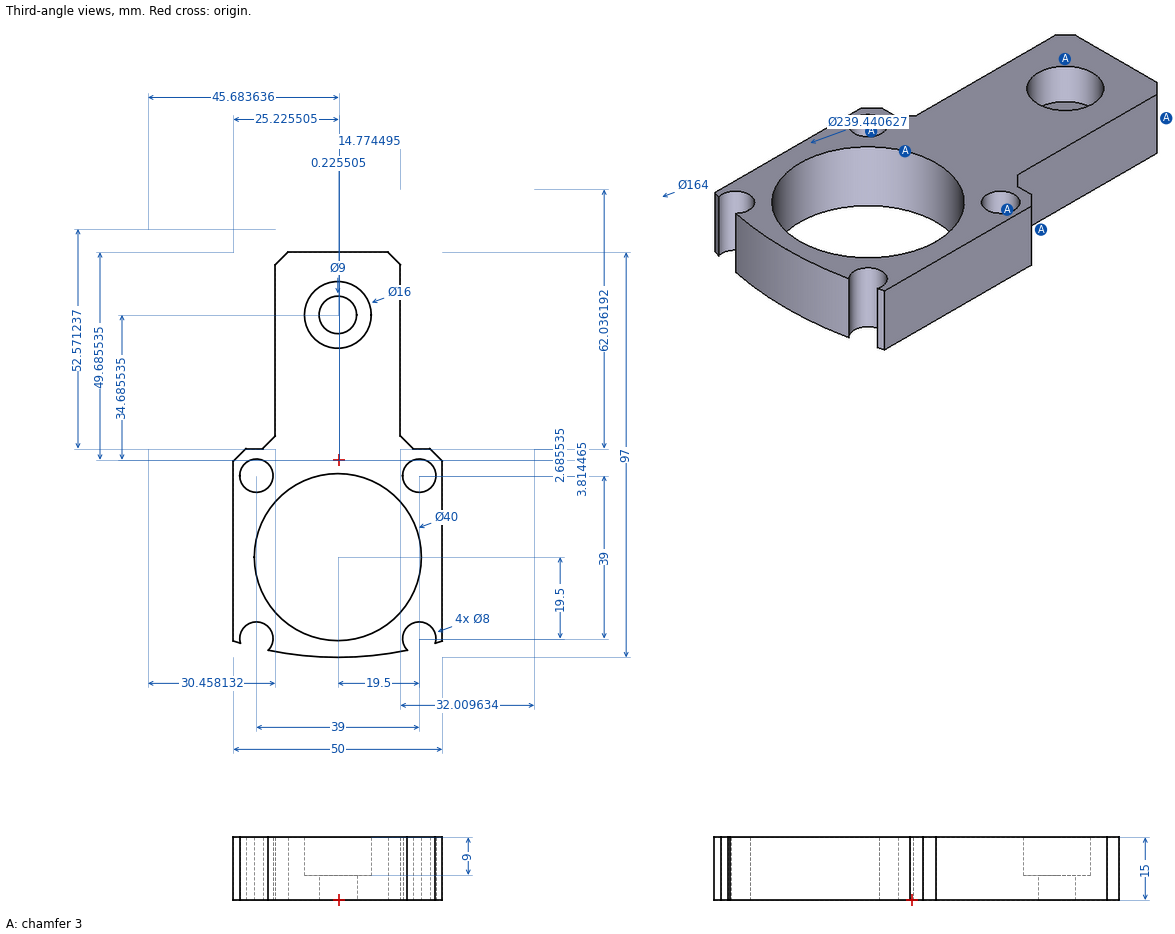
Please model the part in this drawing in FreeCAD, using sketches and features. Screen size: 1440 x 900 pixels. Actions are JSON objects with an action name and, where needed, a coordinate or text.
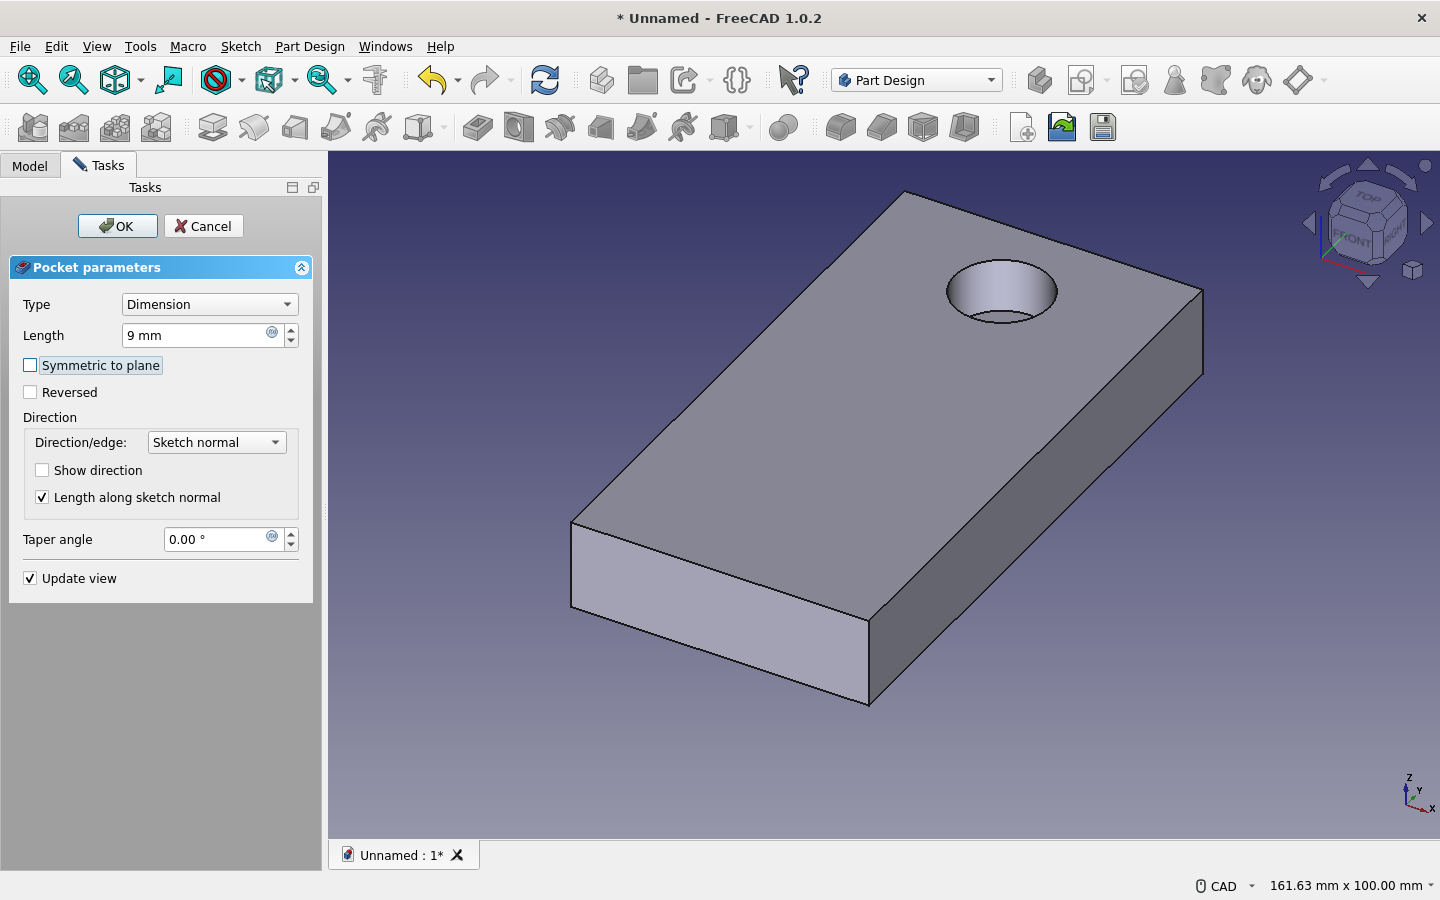
{"action": "left_click", "coordinate": [118, 226]}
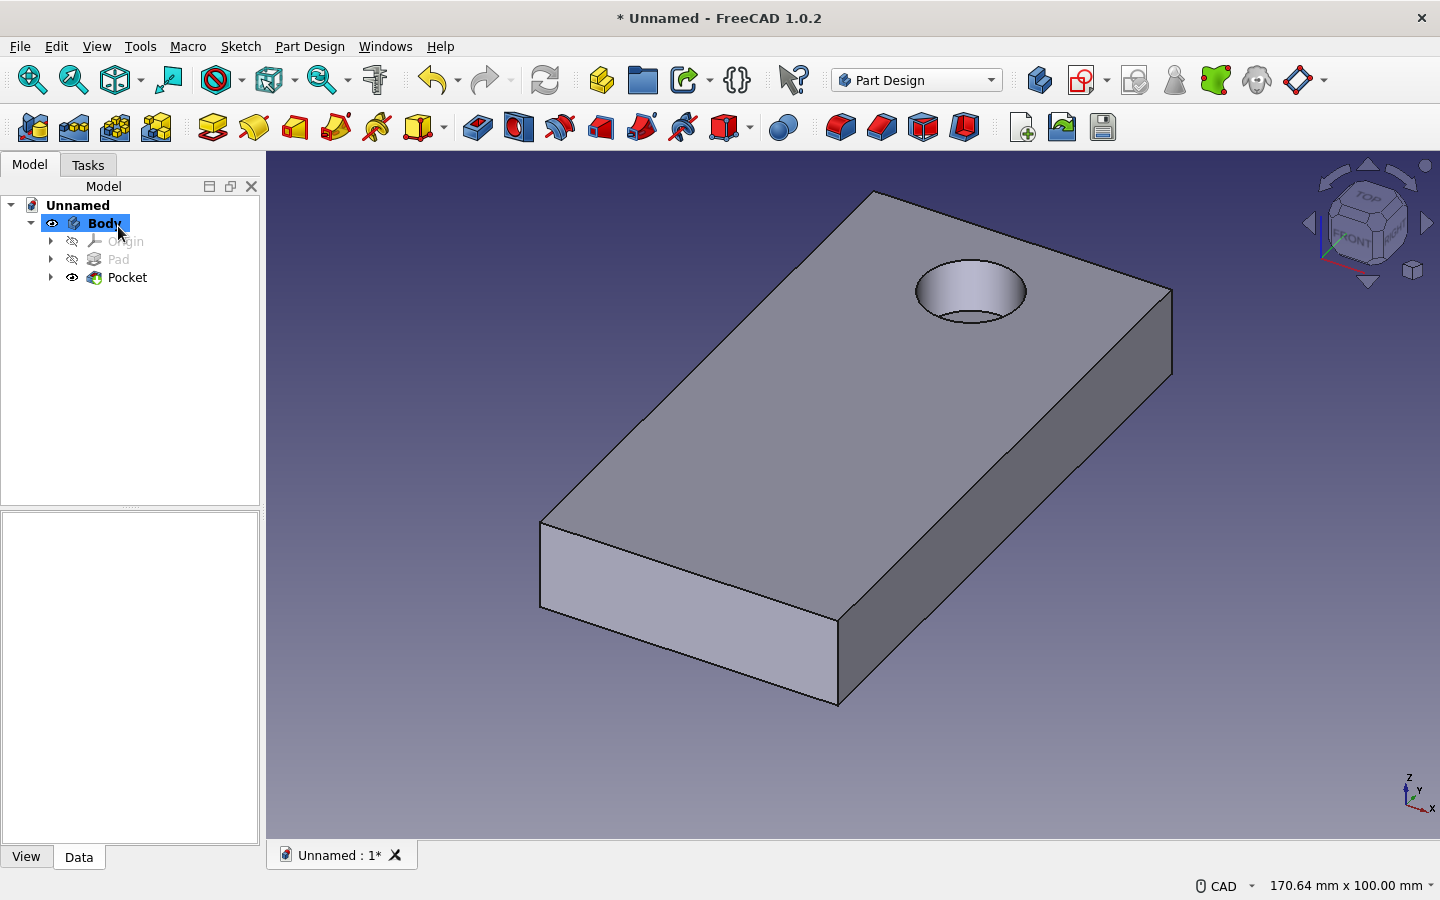
{"action": "key", "text": "0"}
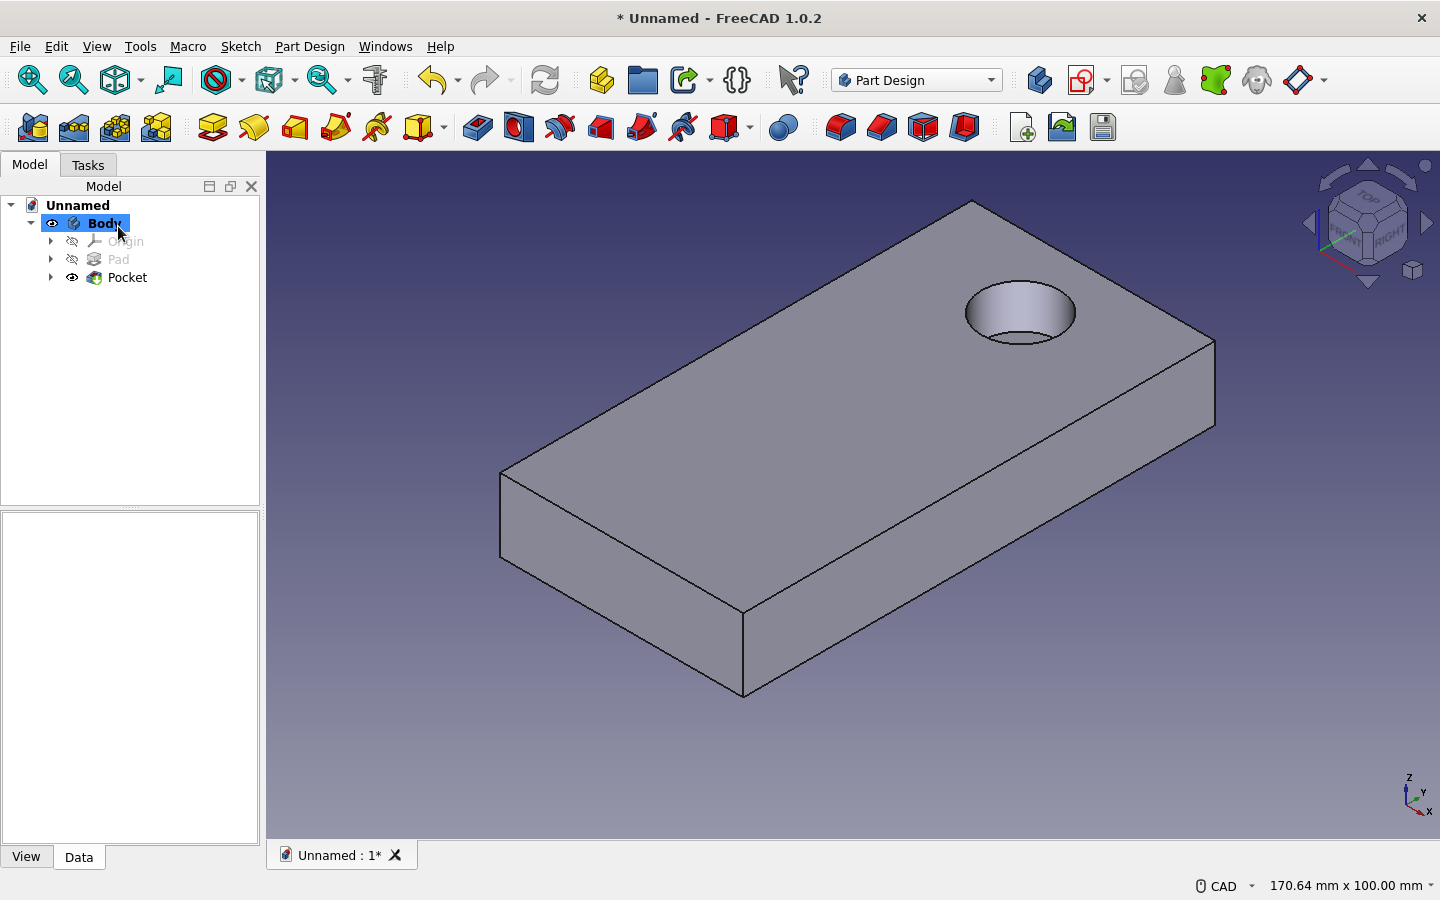
{"action": "key", "text": "2"}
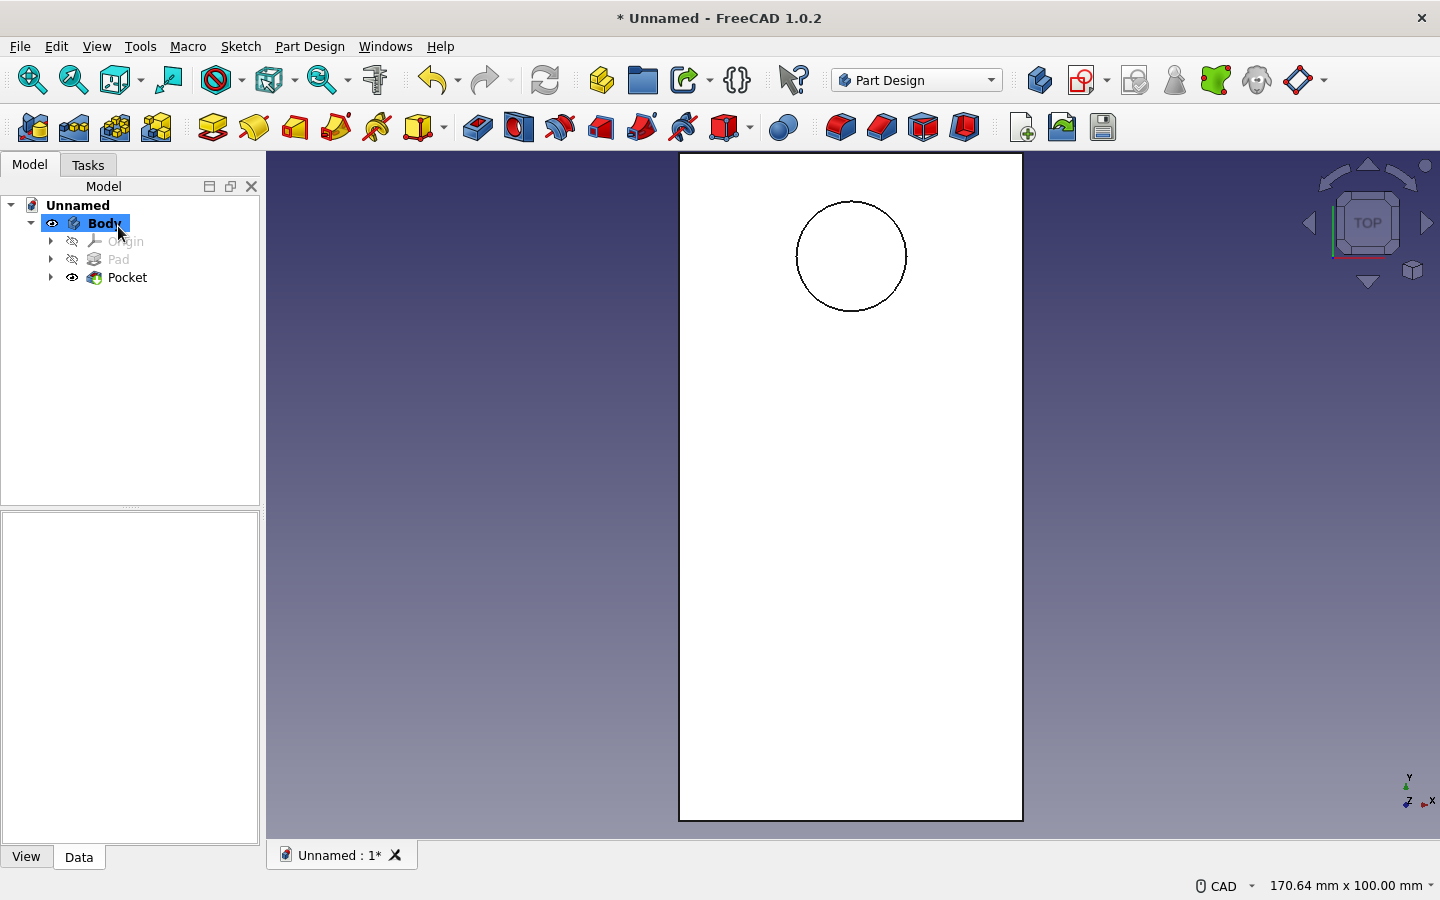
{"action": "left_click", "coordinate": [851, 255]}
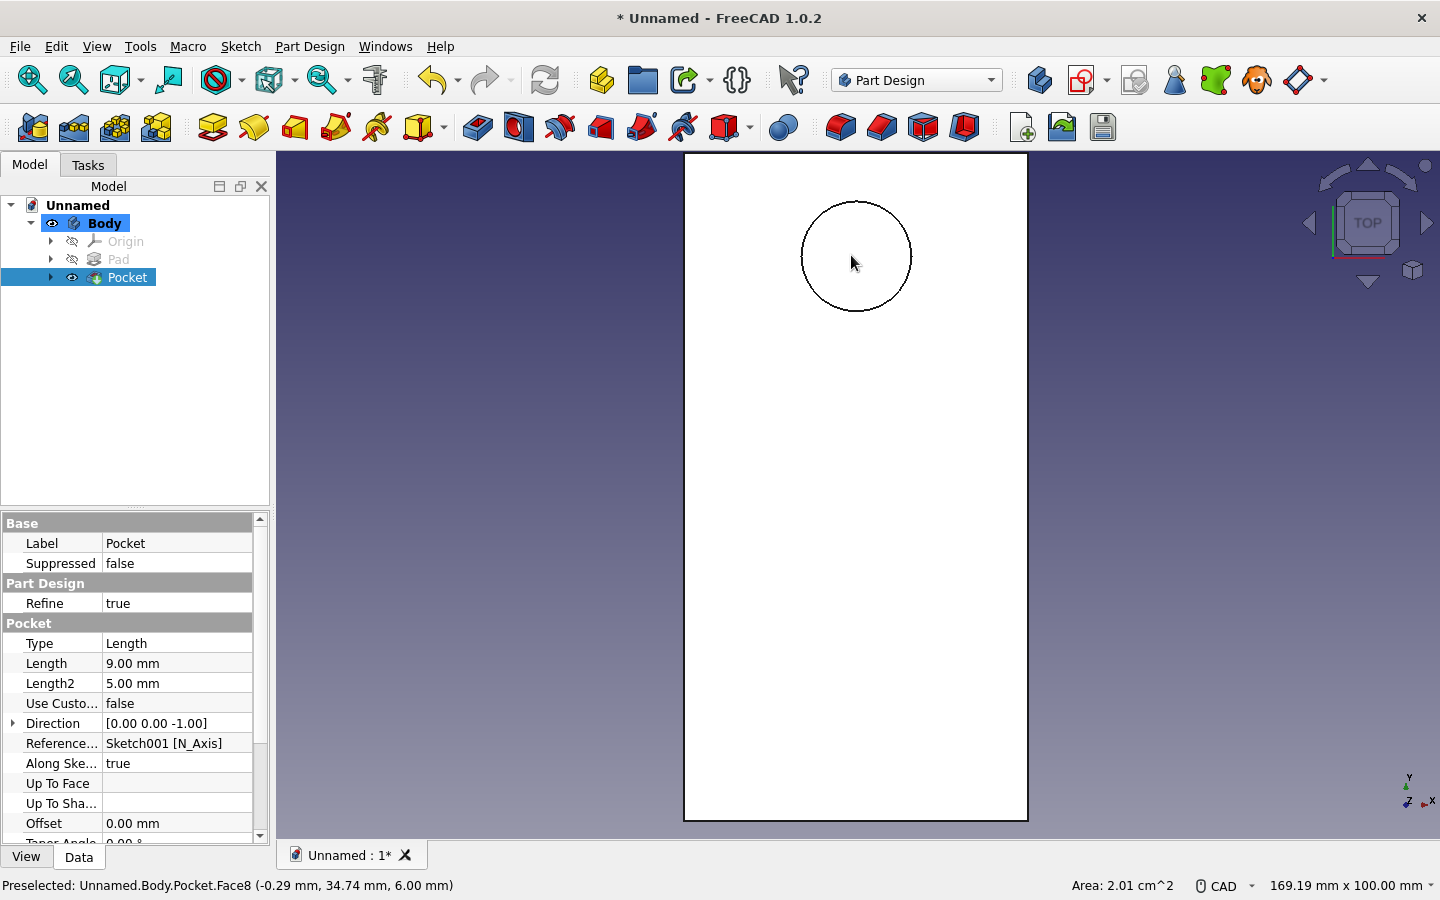
{"action": "left_click", "coordinate": [1080, 80]}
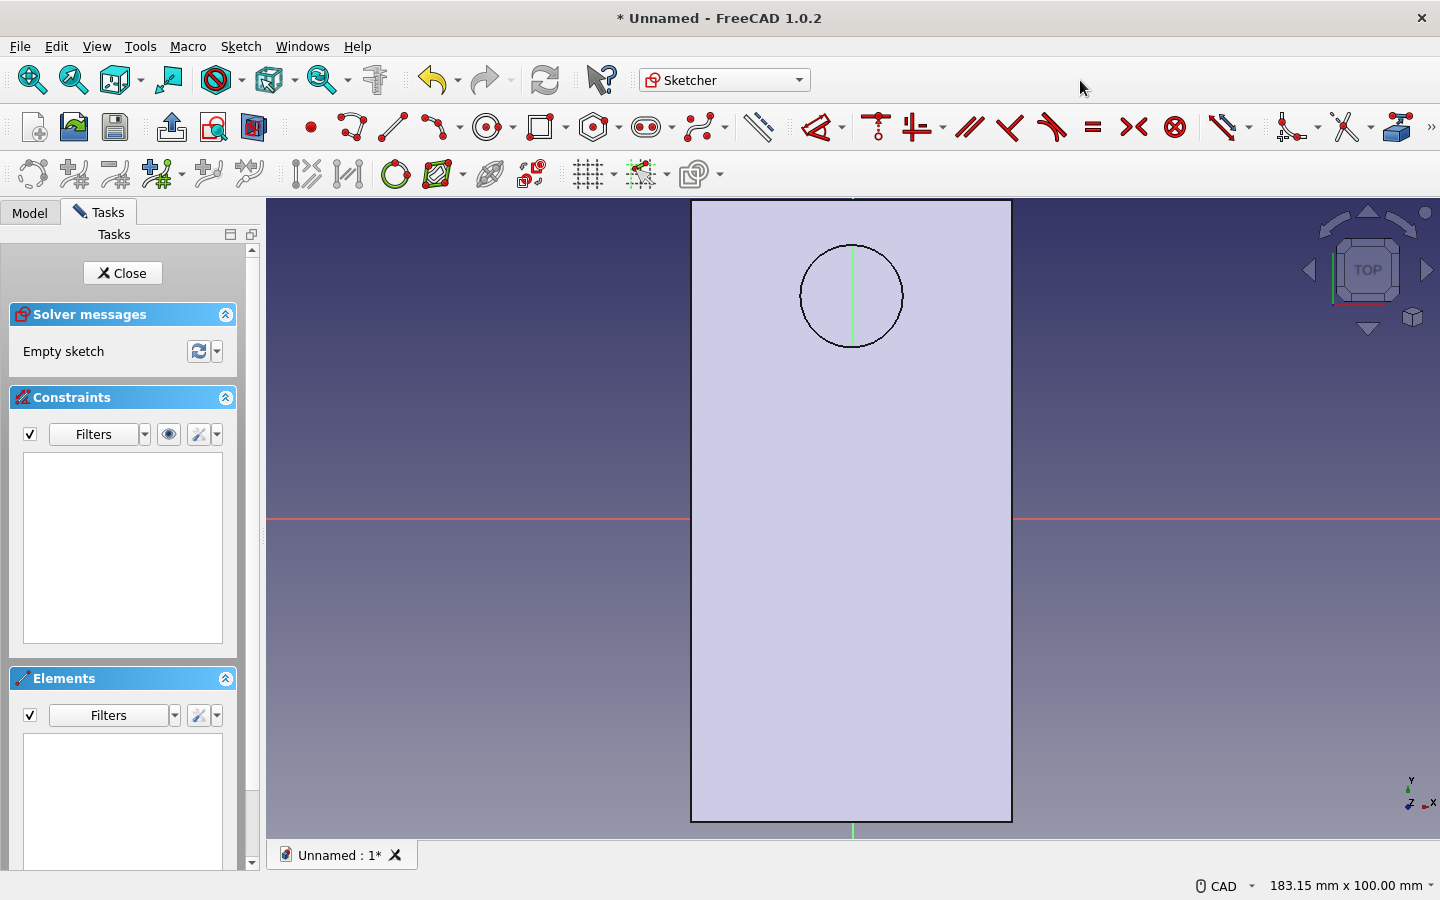
{"action": "key", "text": "q s"}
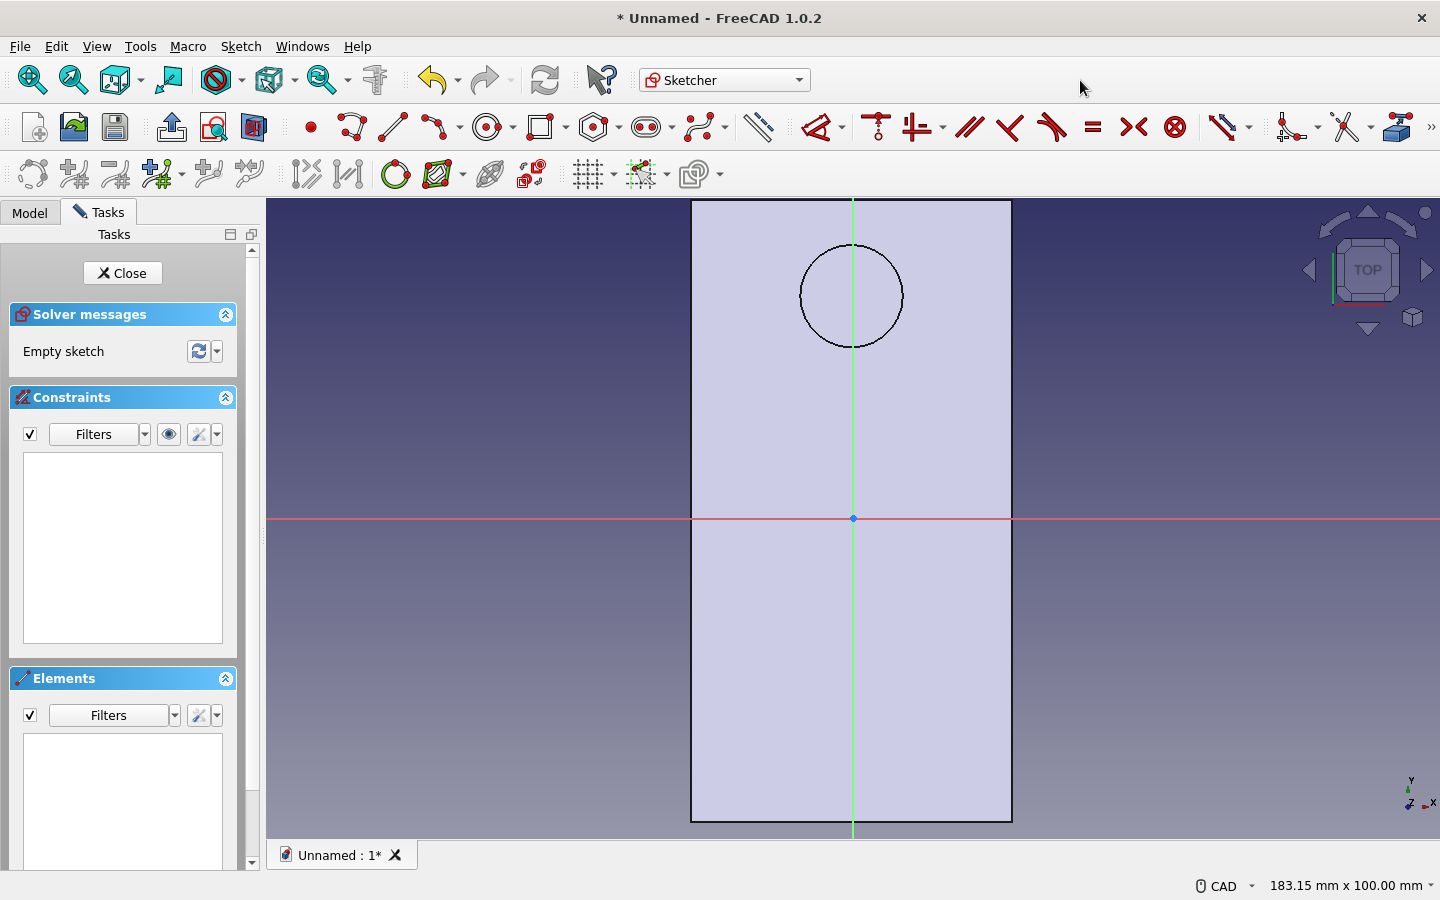
{"action": "scroll", "coordinate": [862, 261], "scroll_direction": "up", "scroll_amount": 10}